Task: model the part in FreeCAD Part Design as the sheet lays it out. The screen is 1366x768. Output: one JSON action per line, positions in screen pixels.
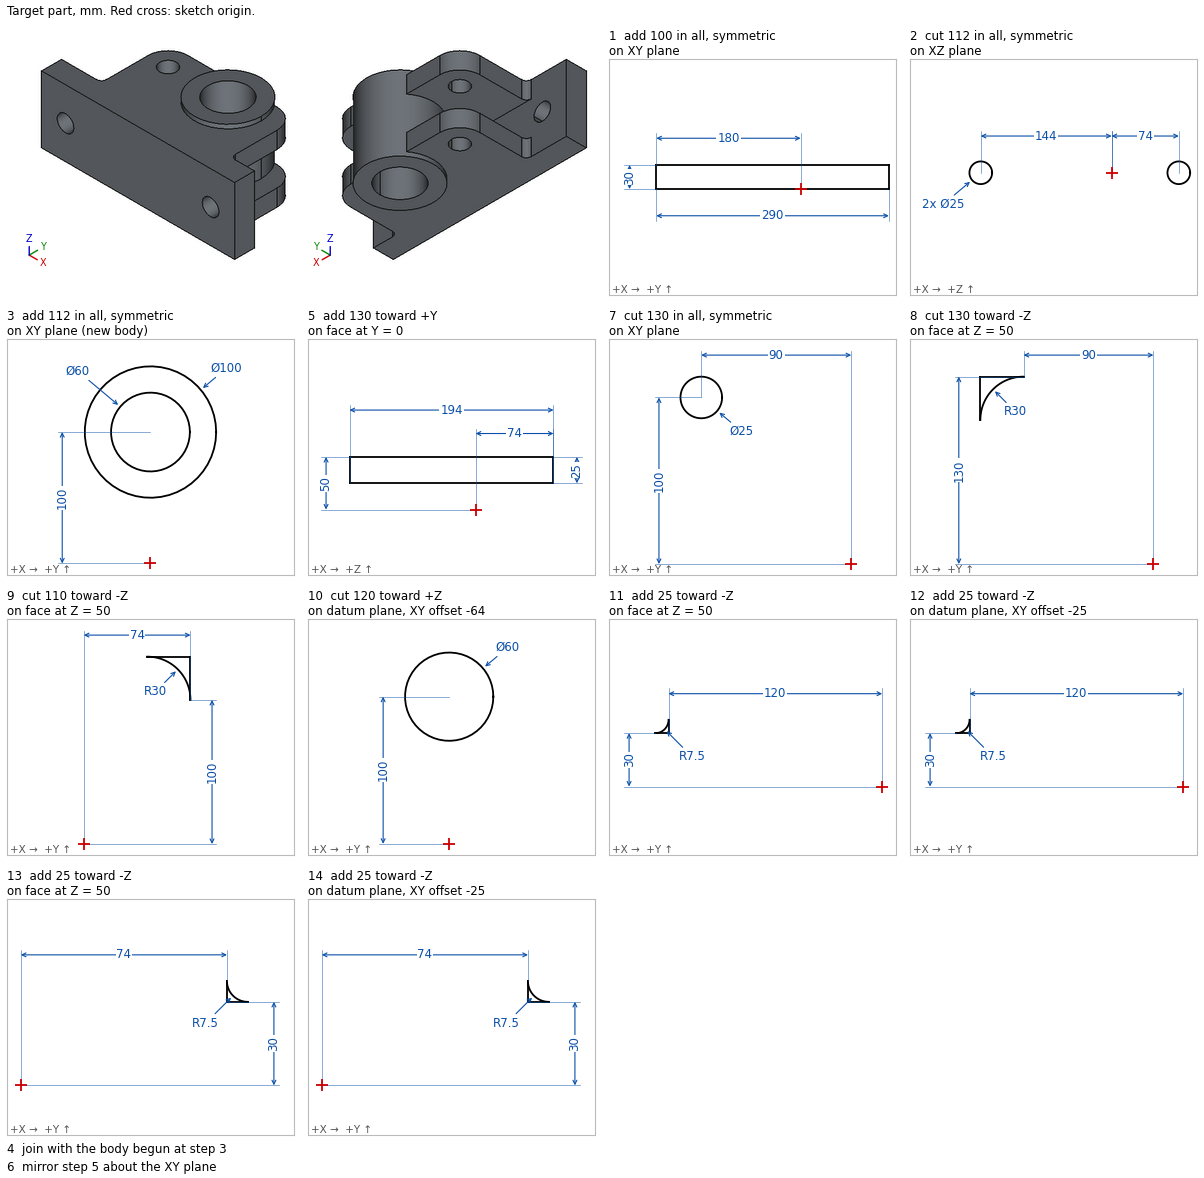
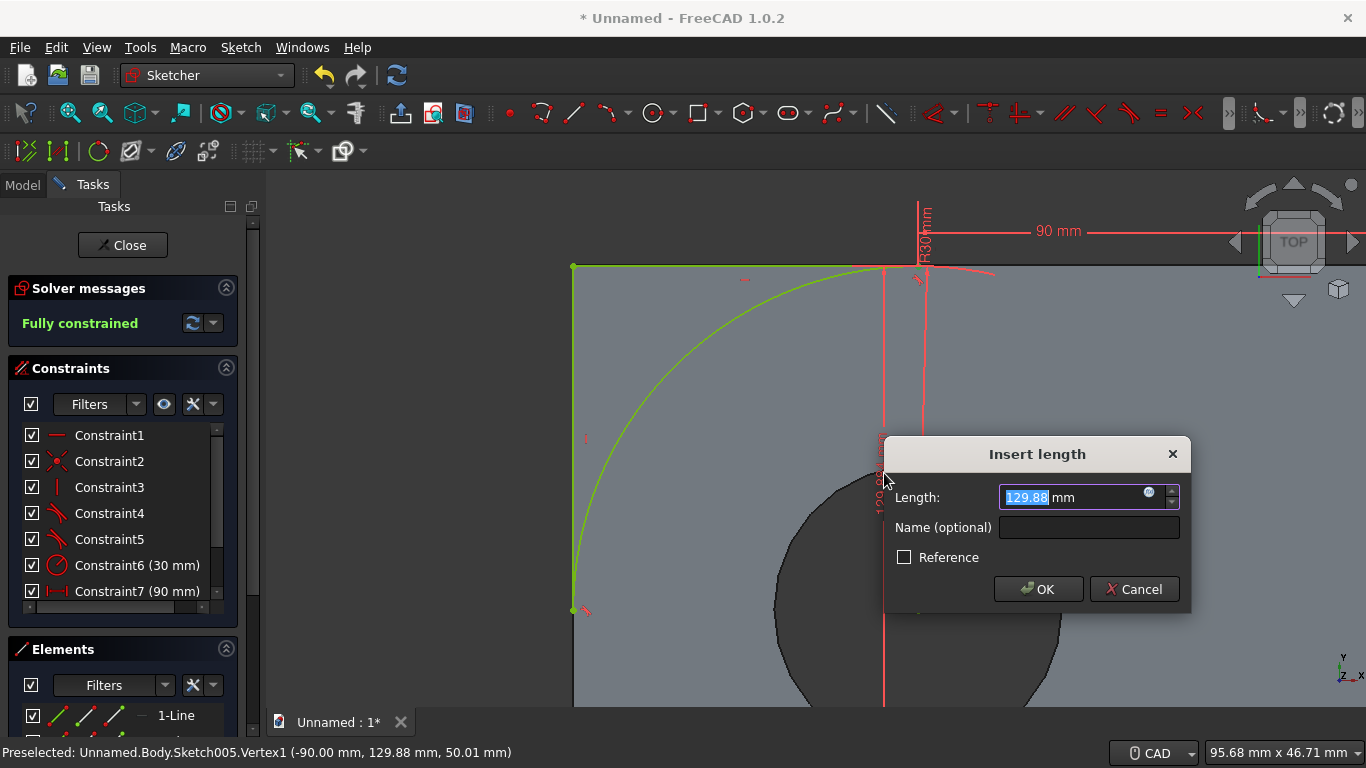
{"action": "type", "text": "130"}
{"action": "key", "text": "Return"}
{"action": "key", "text": "Escape"}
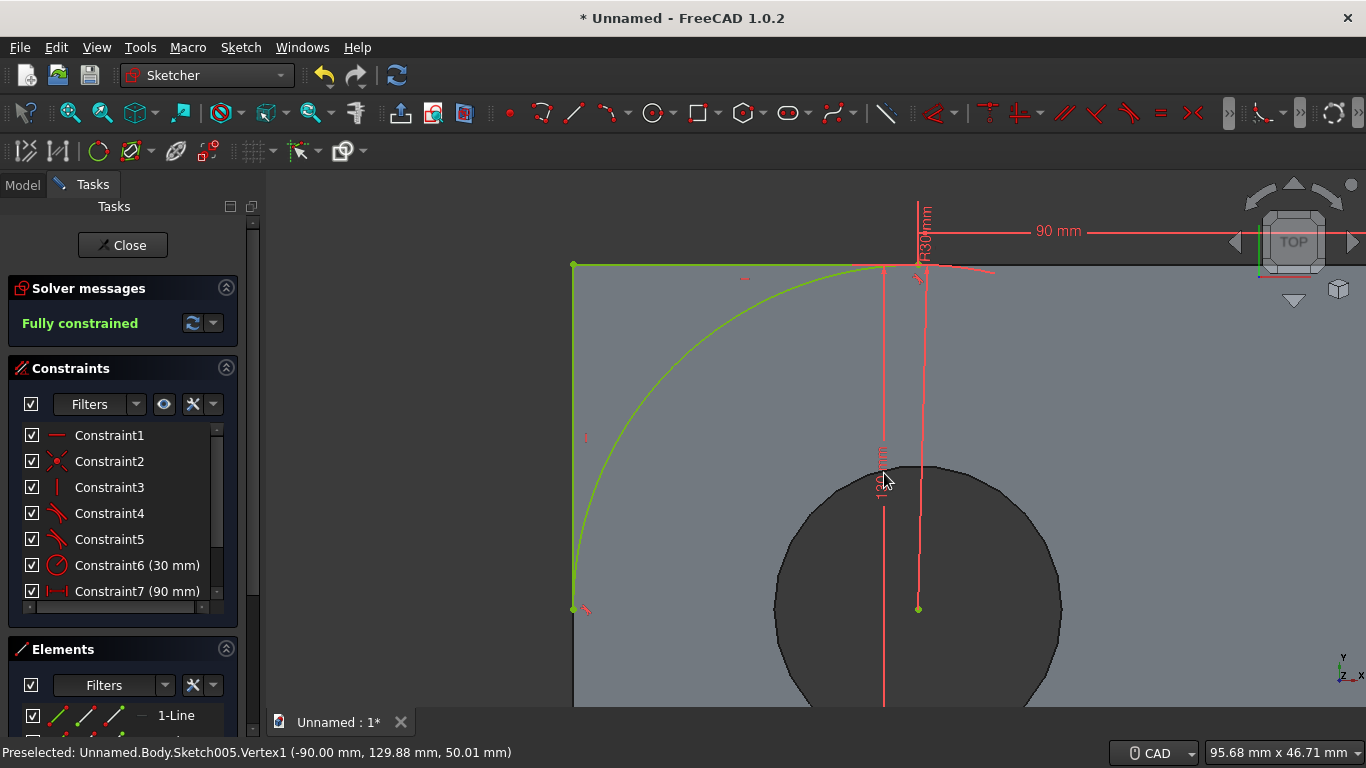
{"action": "left_click", "coordinate": [123, 245]}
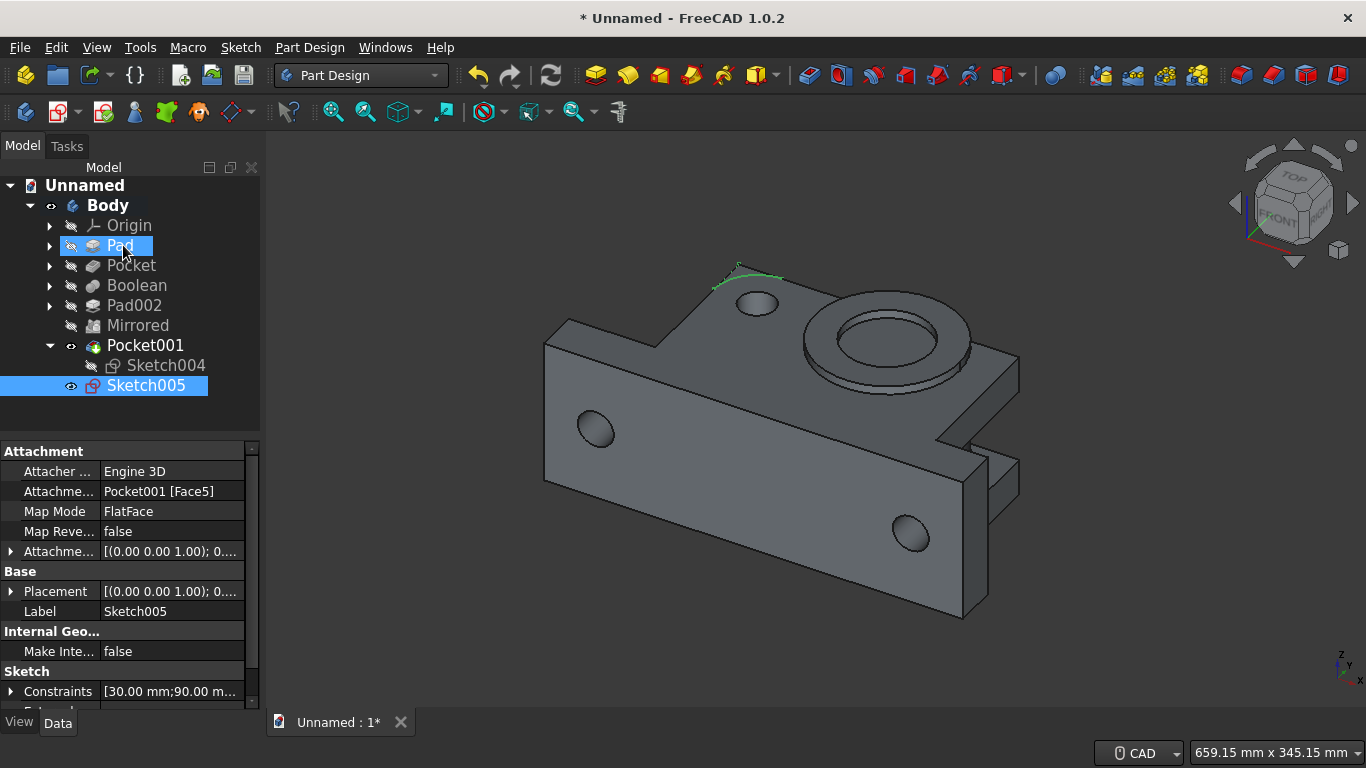
{"action": "left_click", "coordinate": [810, 76]}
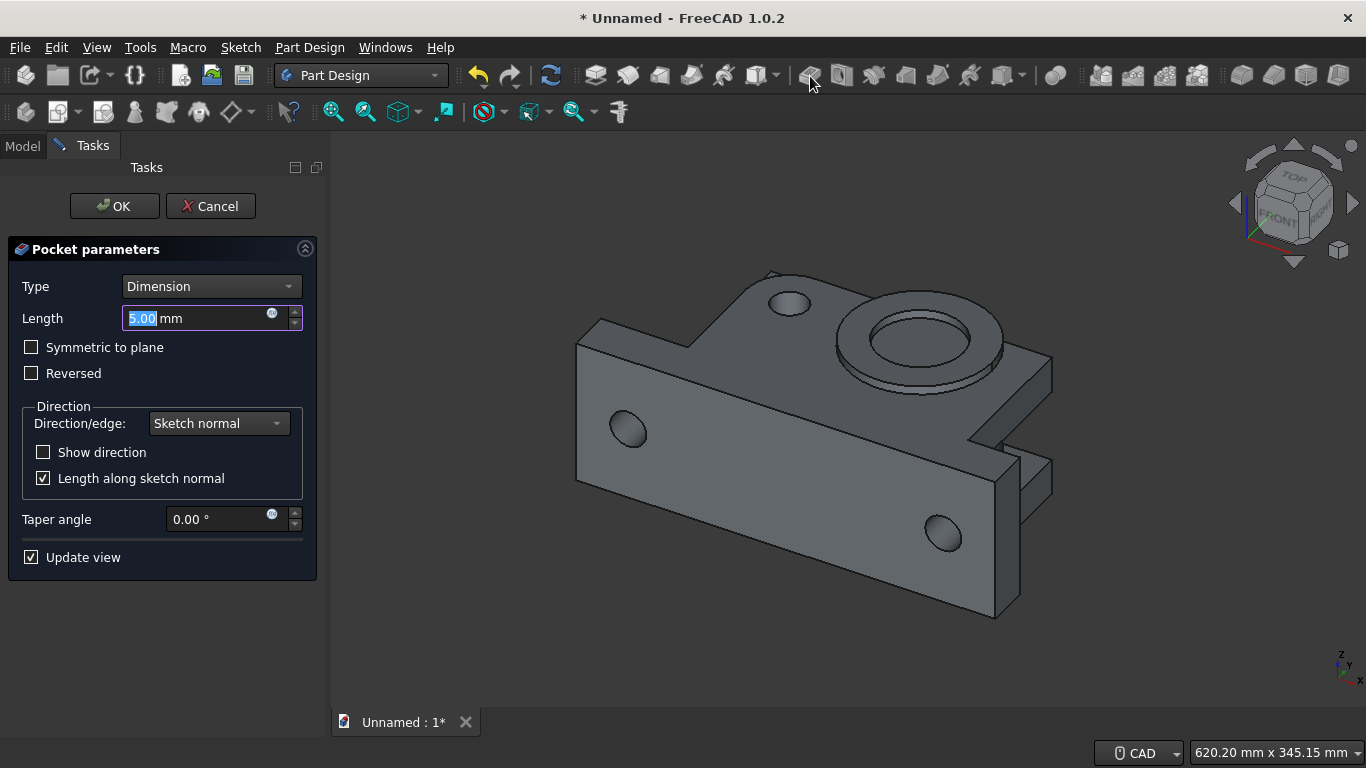
{"action": "type", "text": "130"}
{"action": "key", "text": "Tab"}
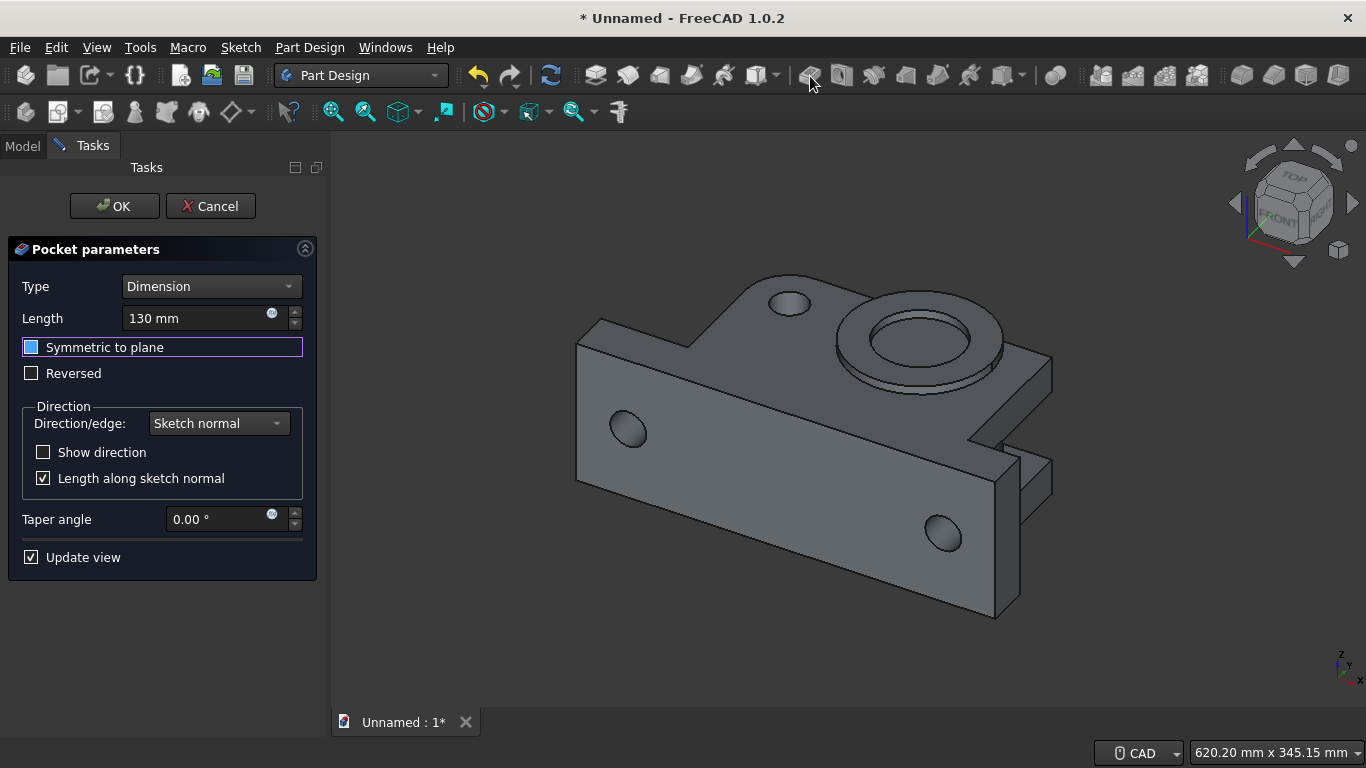
{"action": "left_click", "coordinate": [115, 206]}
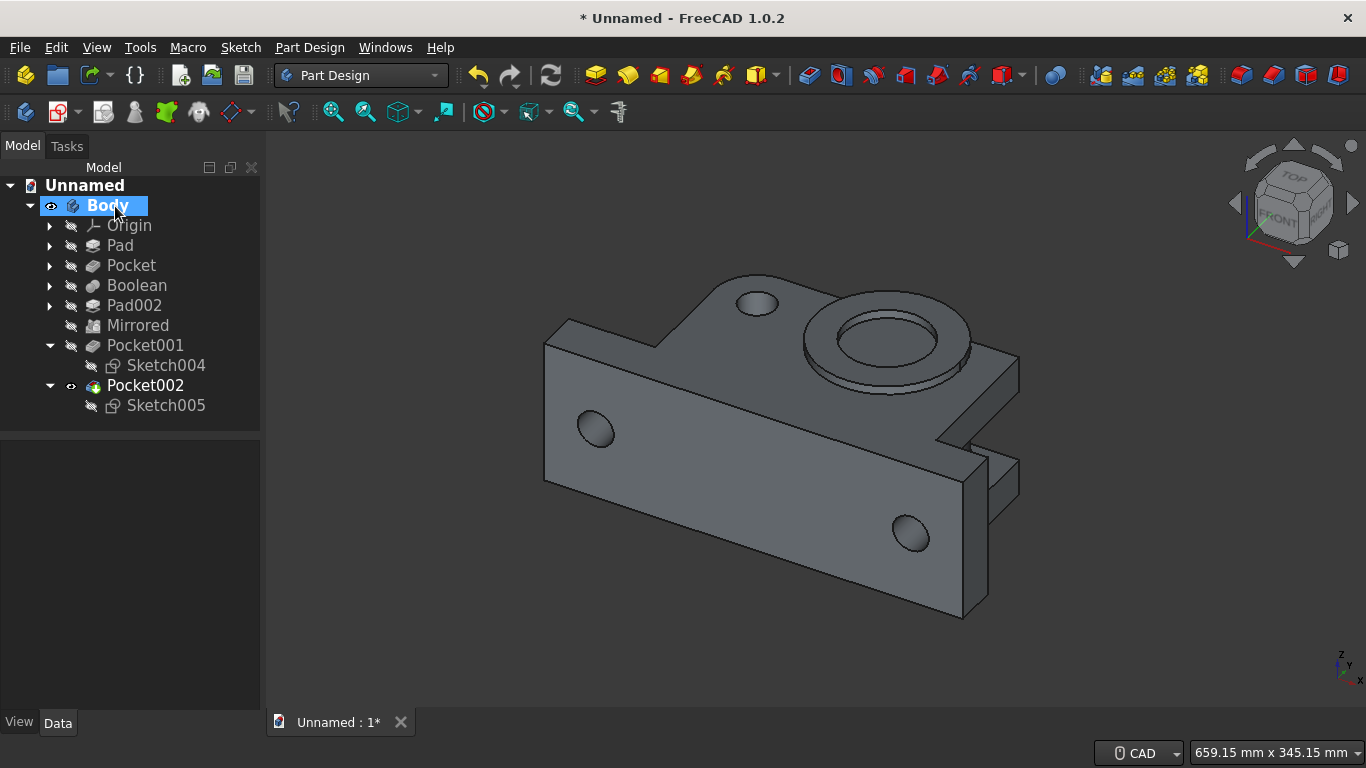
{"action": "left_click", "coordinate": [732, 354]}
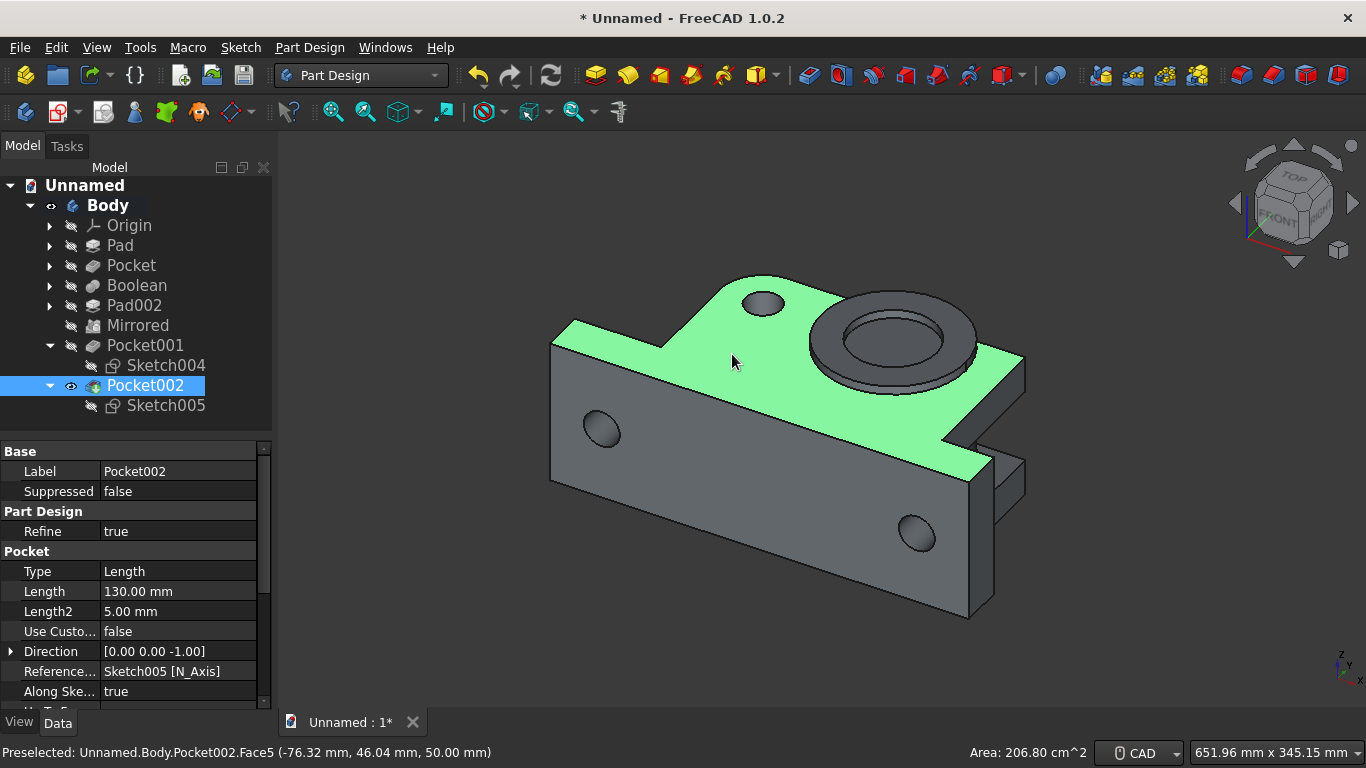
{"action": "left_click", "coordinate": [58, 112]}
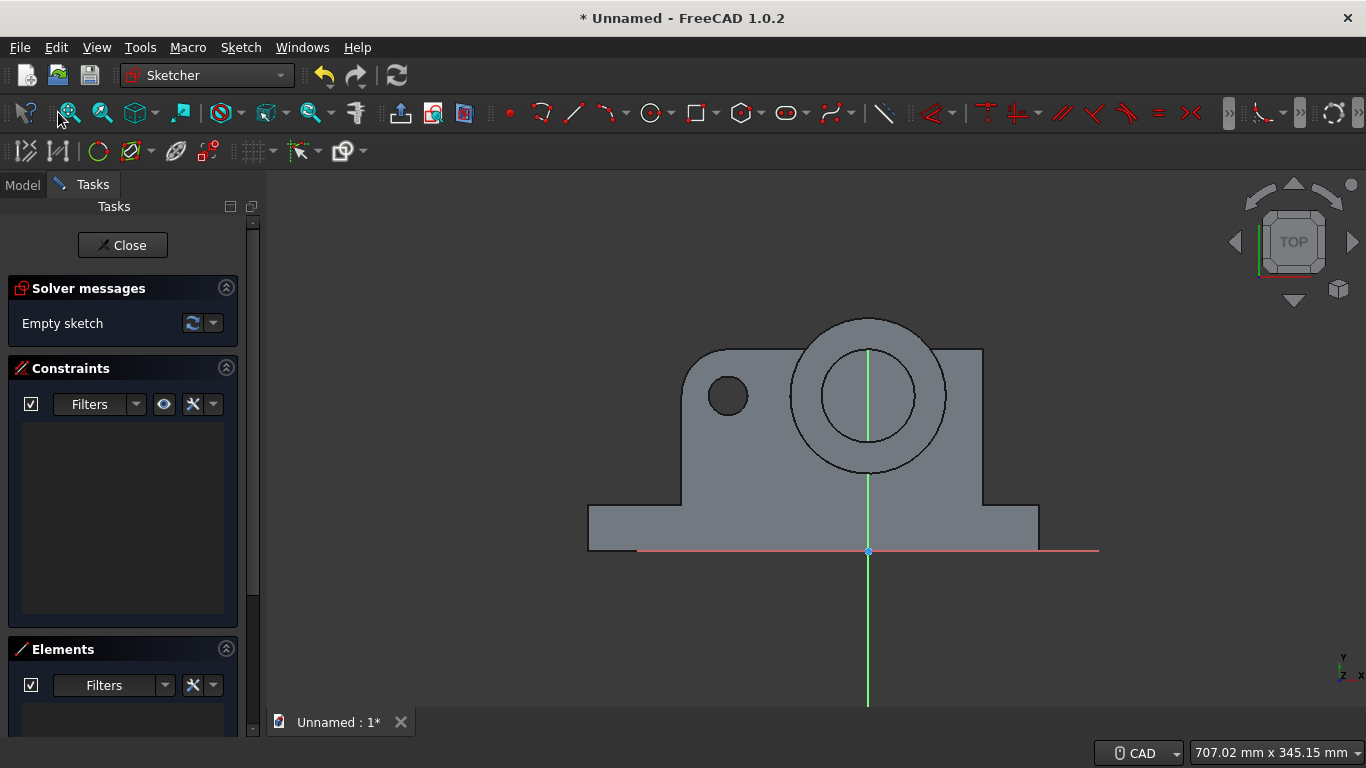
{"action": "left_click", "coordinate": [466, 114]}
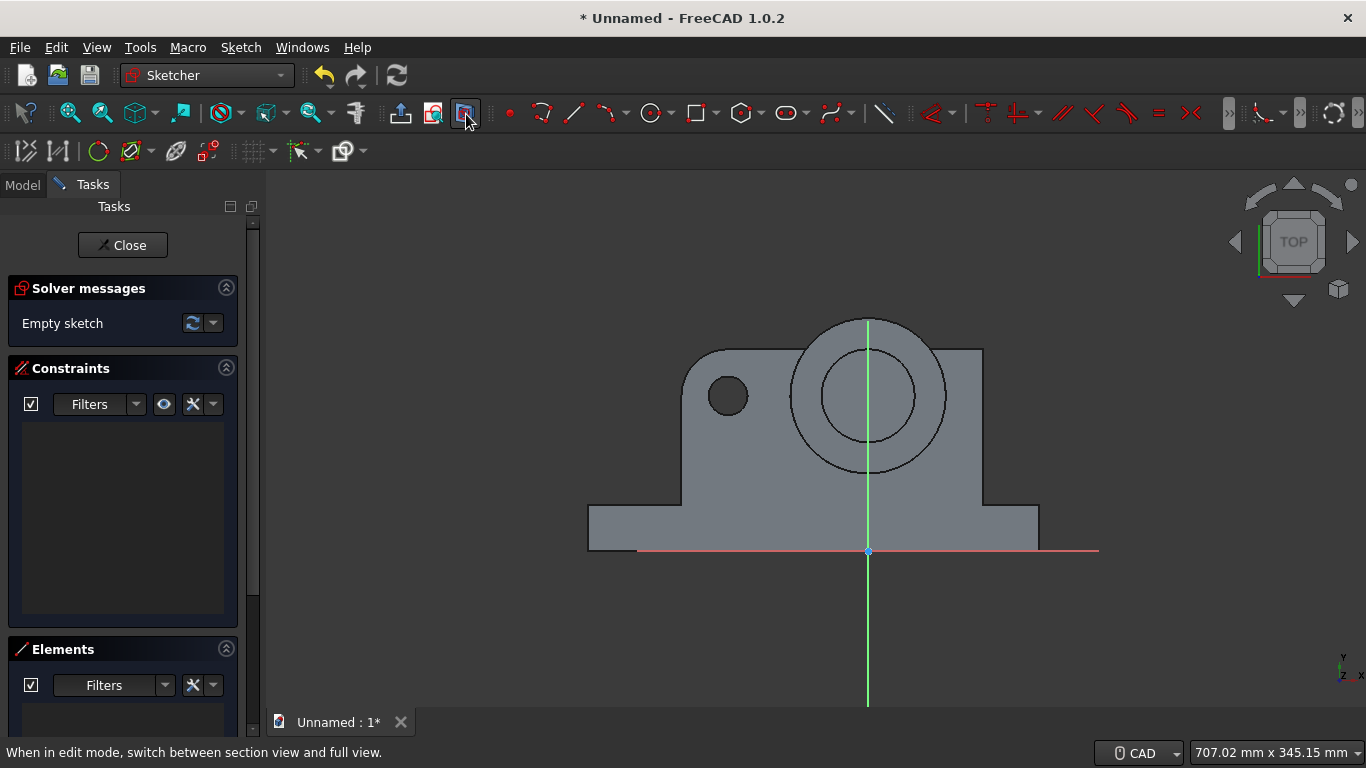
{"action": "scroll", "coordinate": [993, 362], "scroll_direction": "up", "scroll_amount": 10}